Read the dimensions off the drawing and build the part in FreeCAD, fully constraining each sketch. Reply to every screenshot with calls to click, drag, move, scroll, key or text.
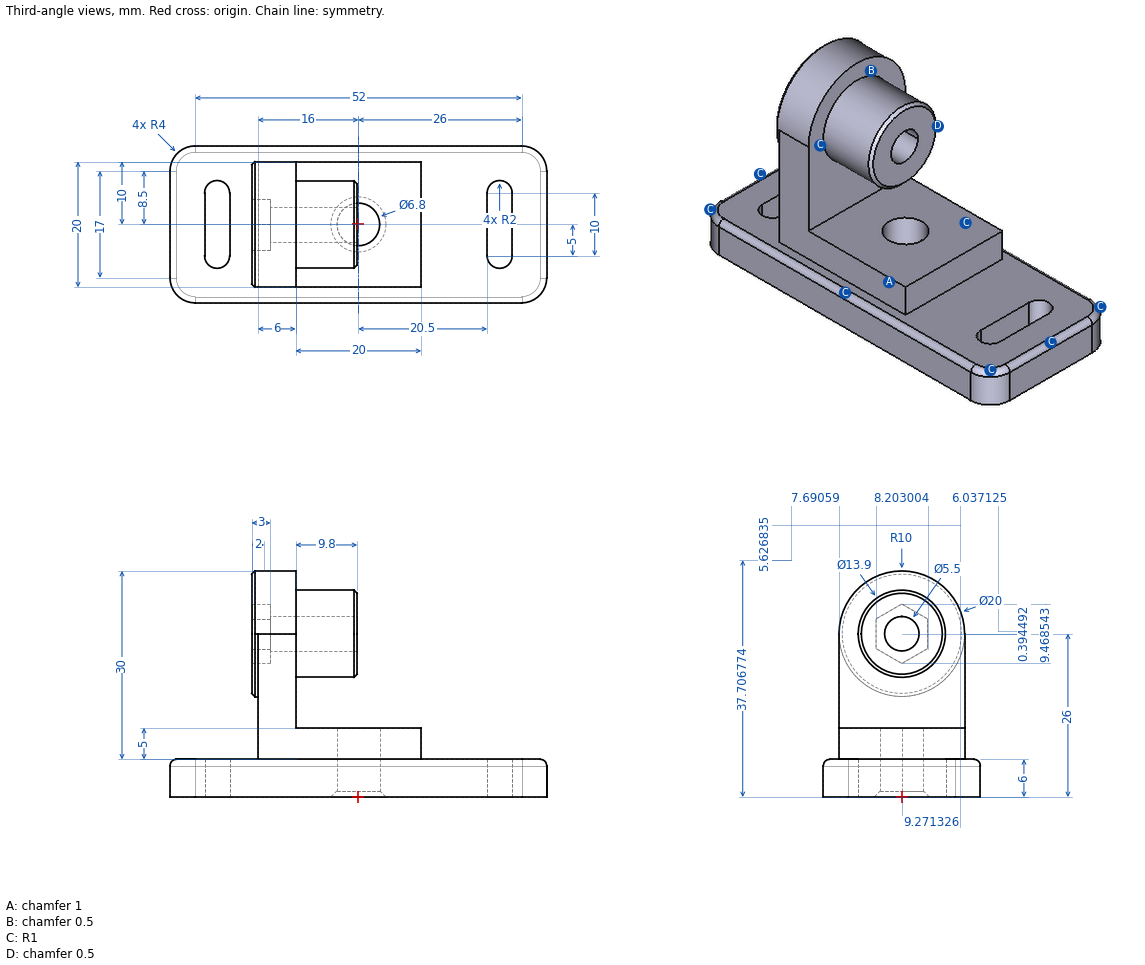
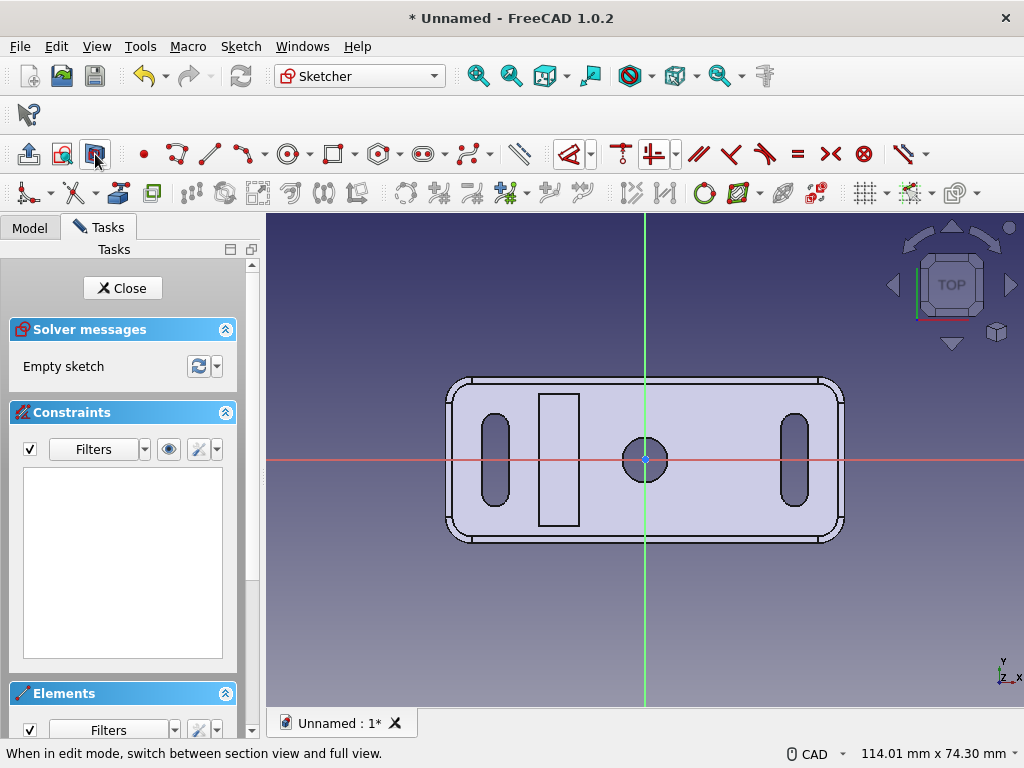
scroll(701, 460, up, 4)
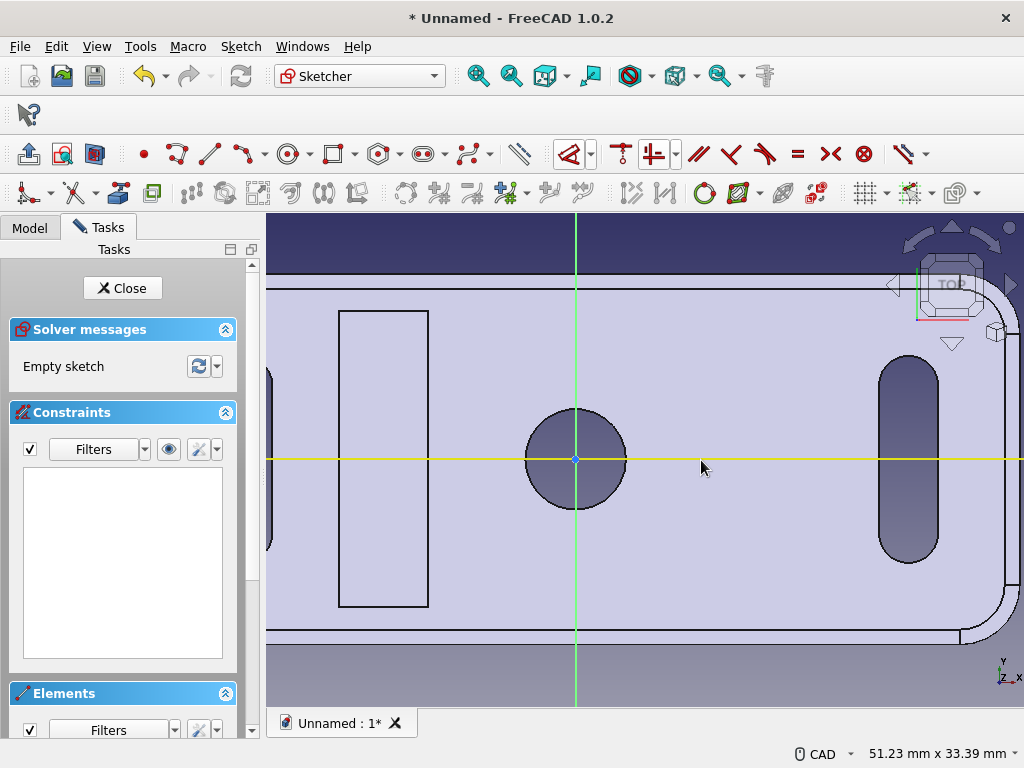
key(g)
key(v)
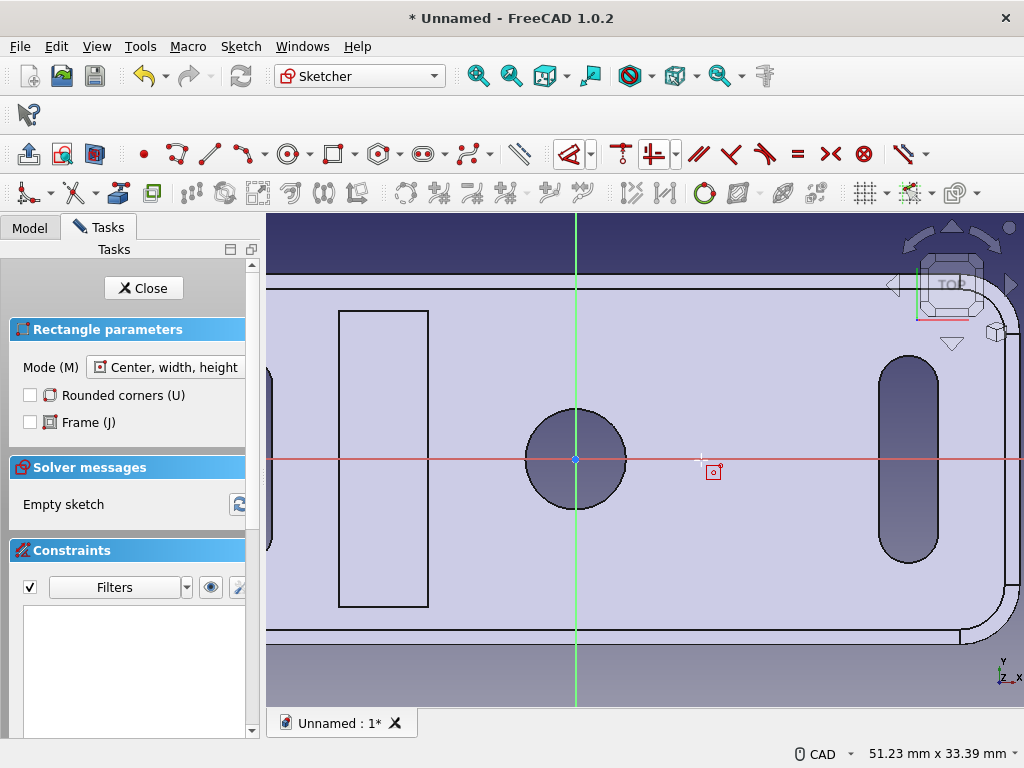
click(576, 459)
move(724, 311)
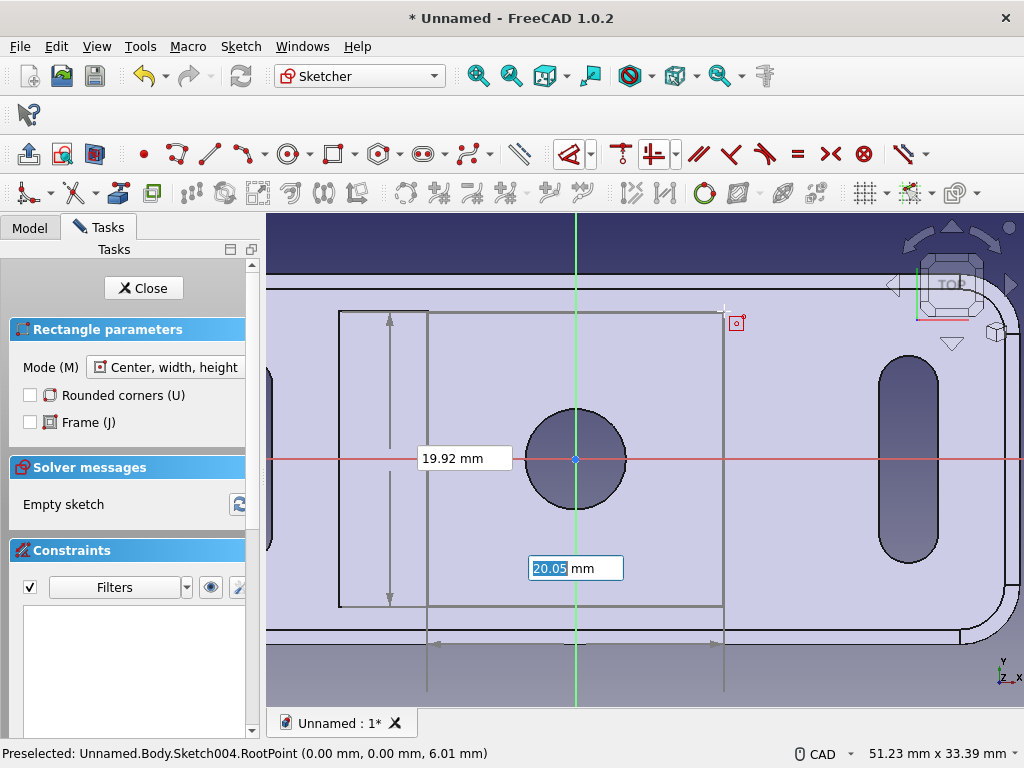
text(20)
key(Tab)
text(20)
key(Return)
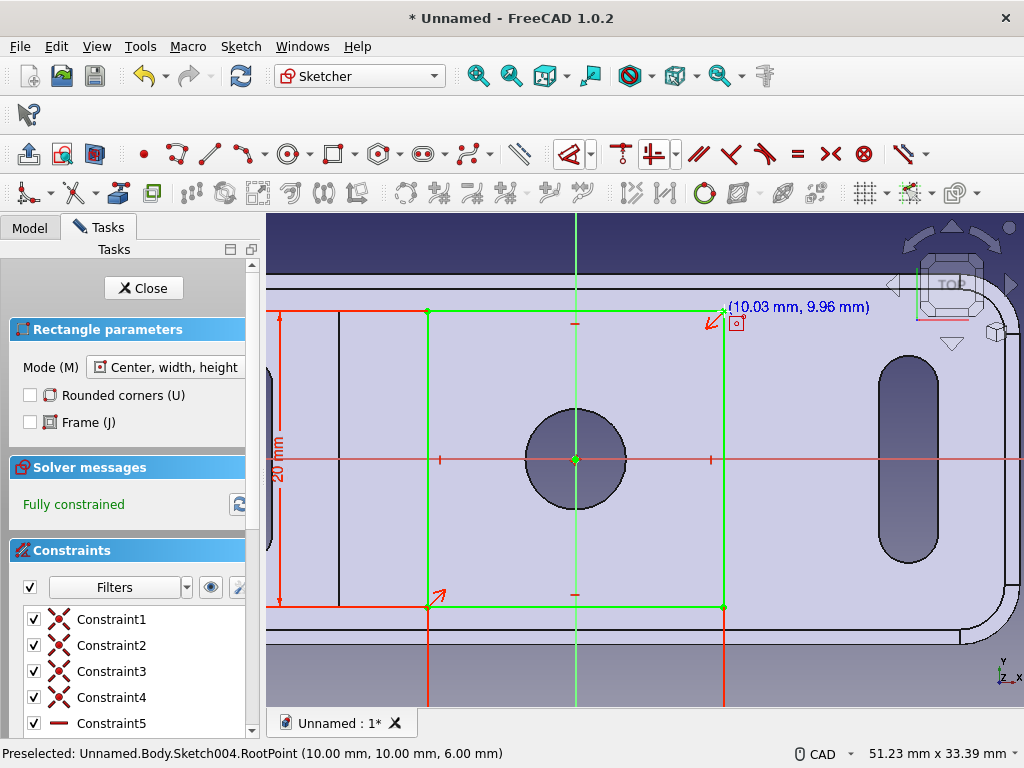
click(288, 154)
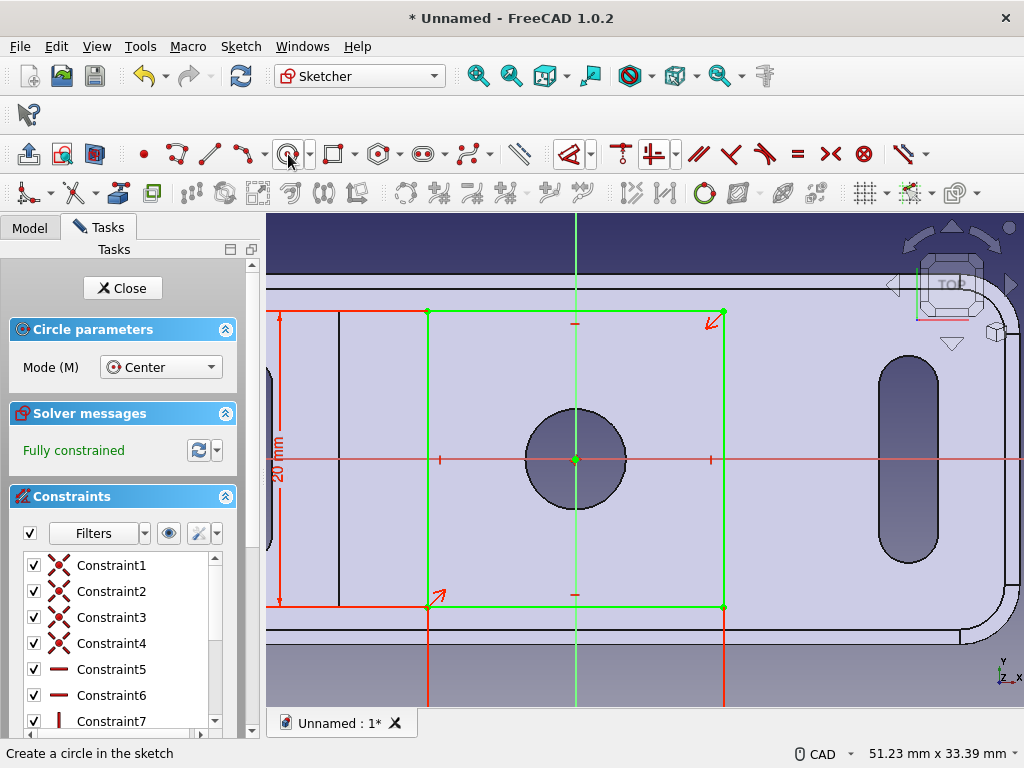
click(576, 459)
move(611, 424)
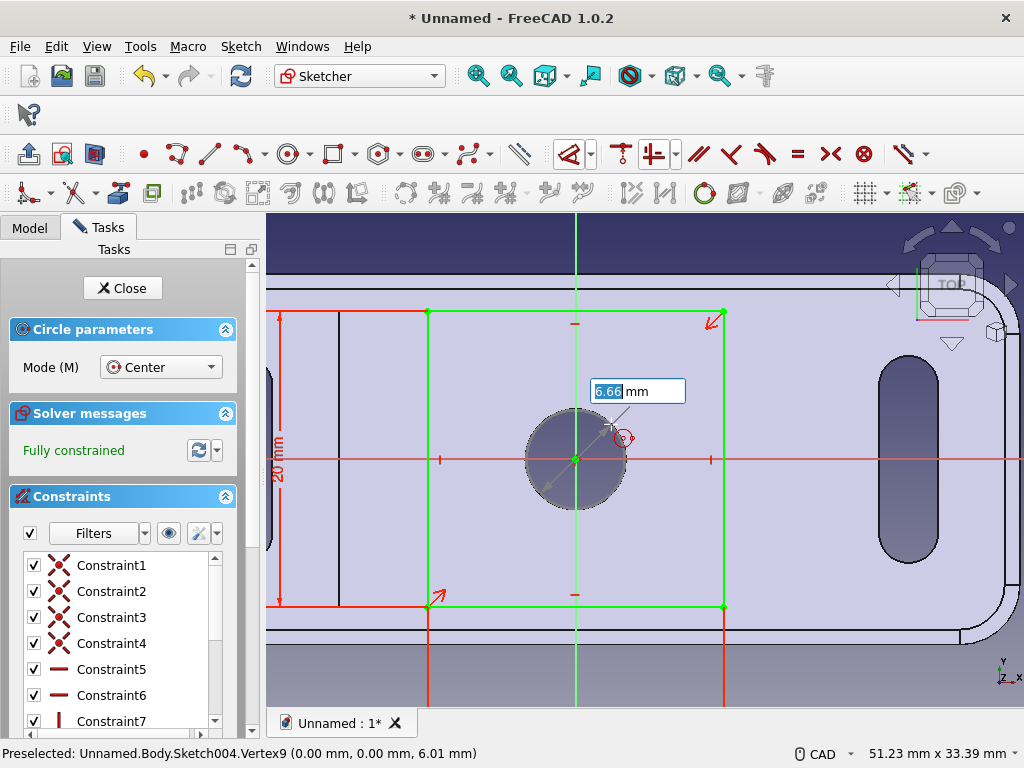
text(6.8)
key(Return)
key(Escape)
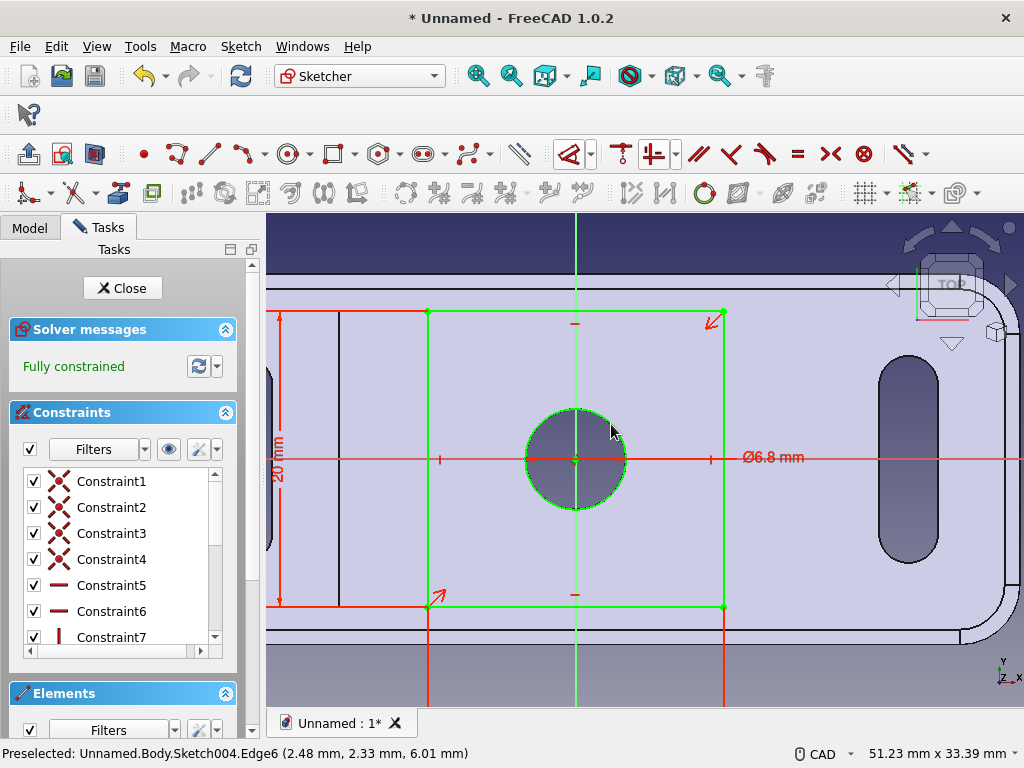
click(123, 288)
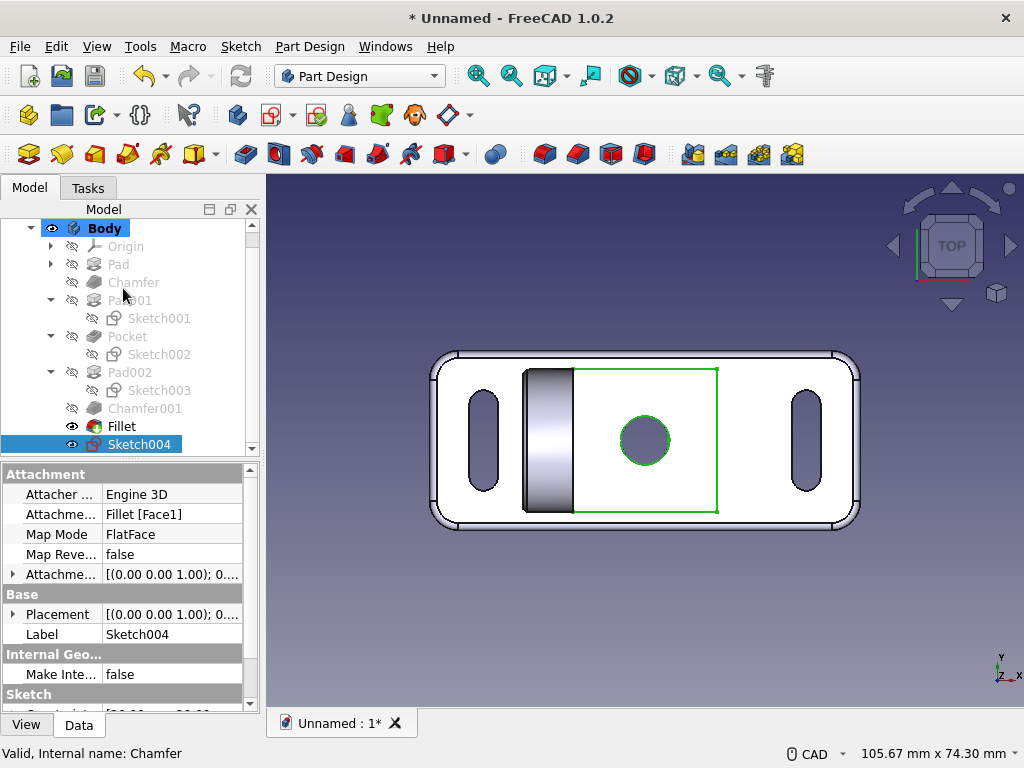
click(29, 154)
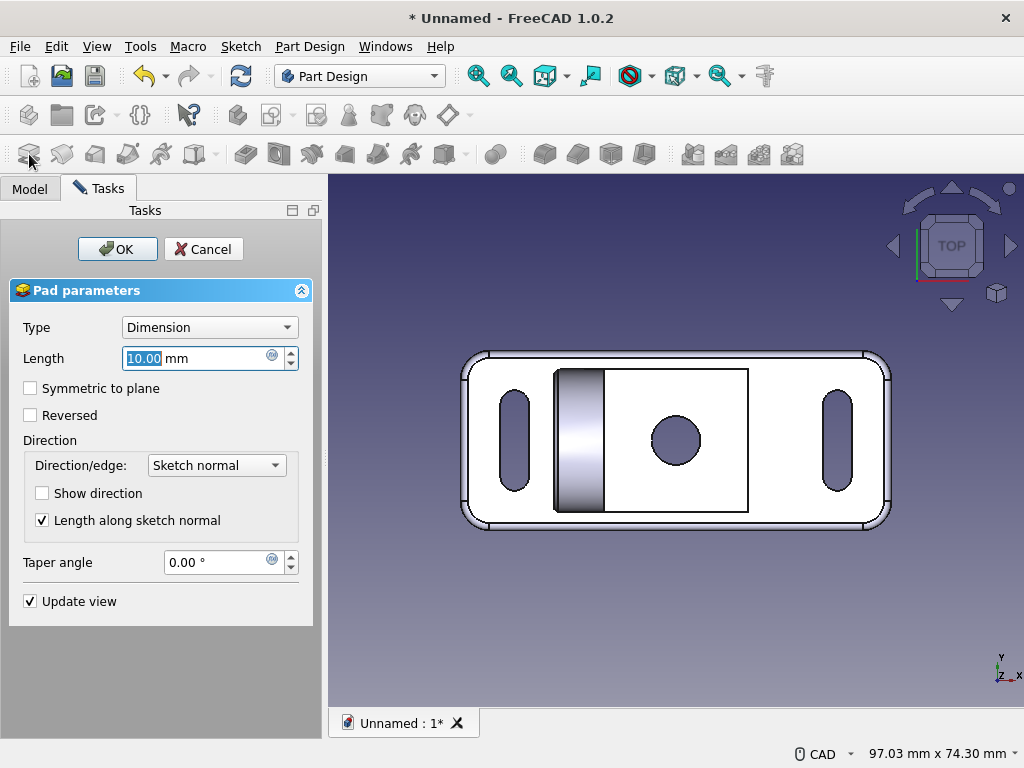
text(5)
key(Tab)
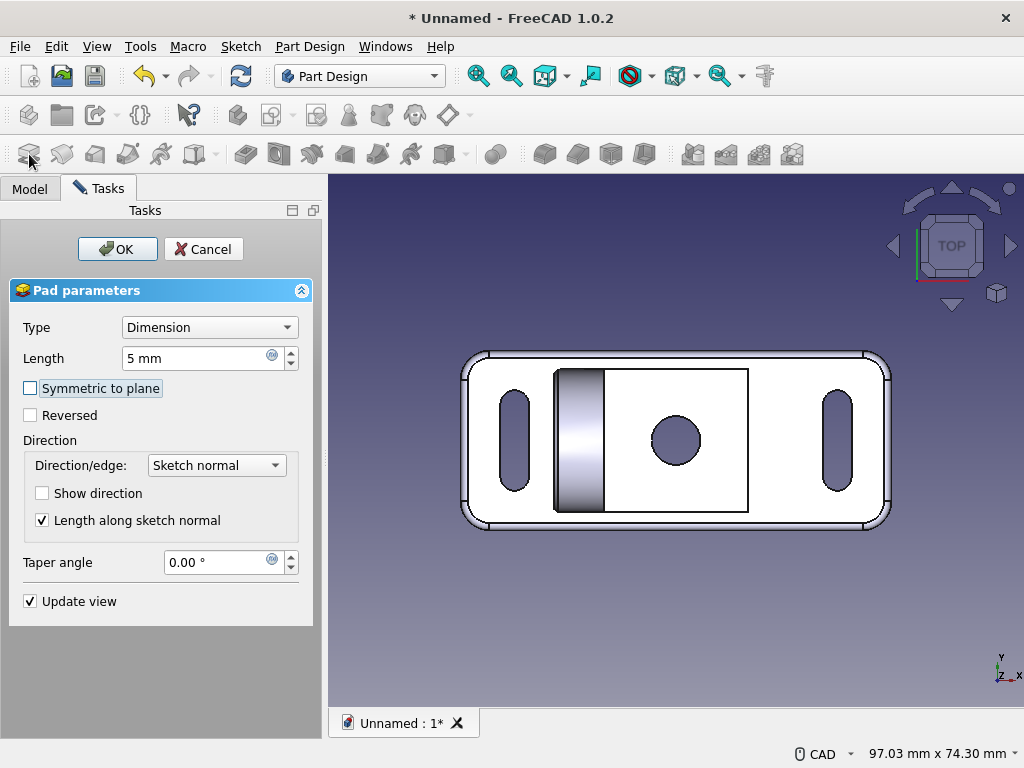
click(118, 249)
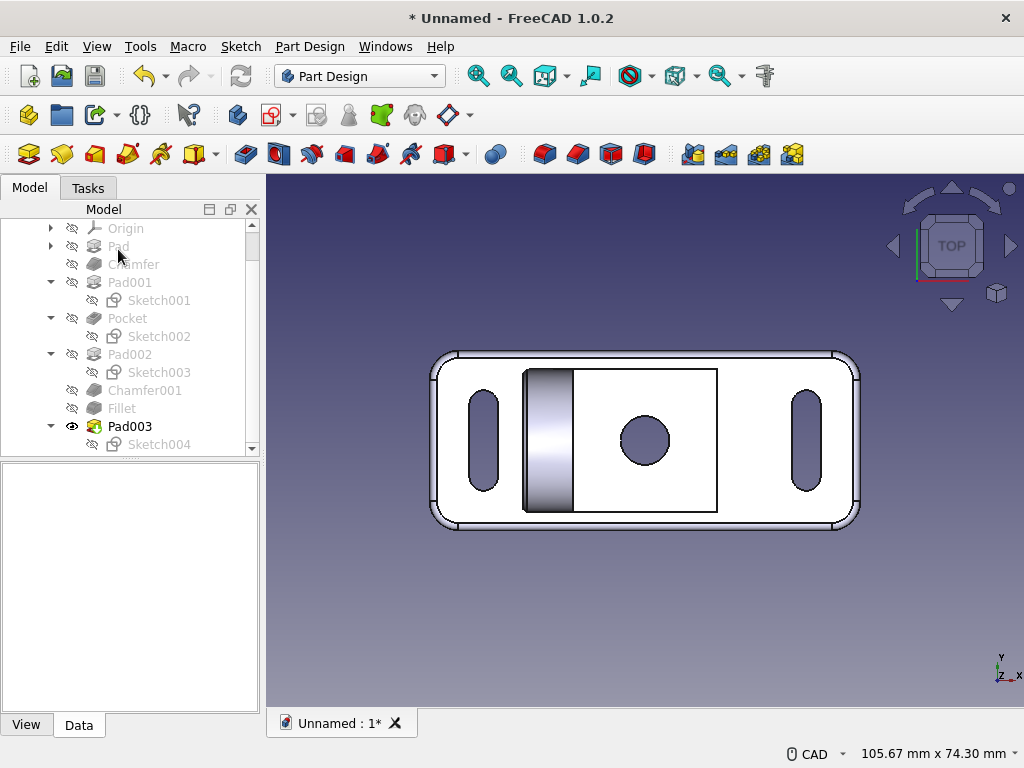
key(6)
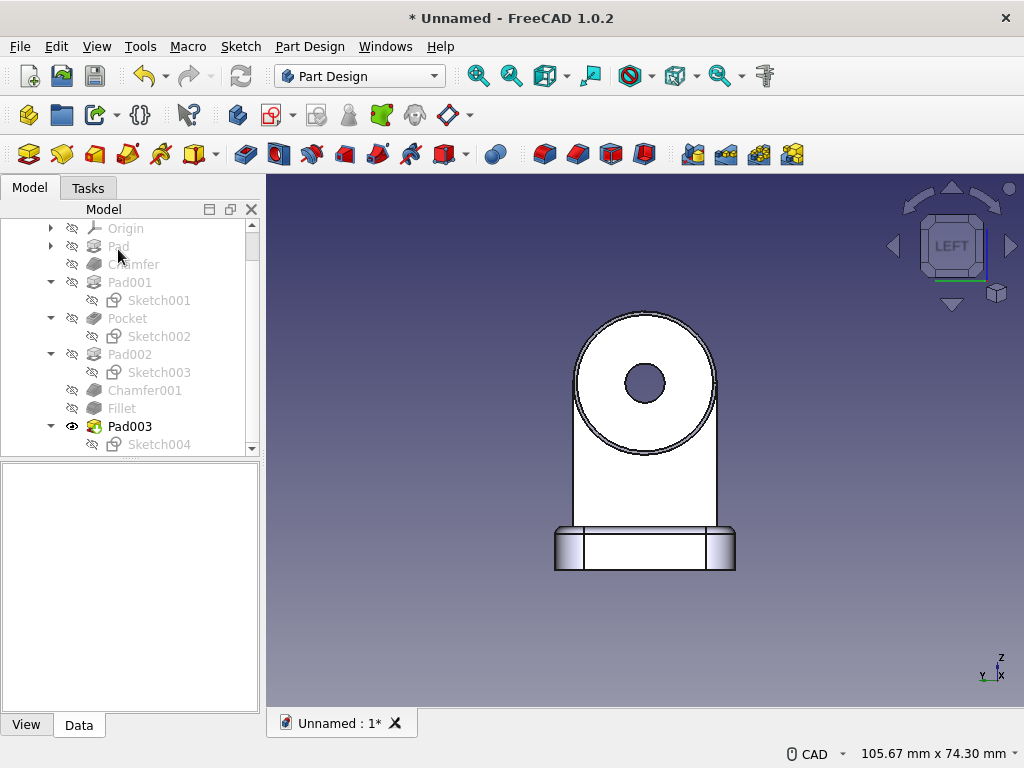
click(626, 421)